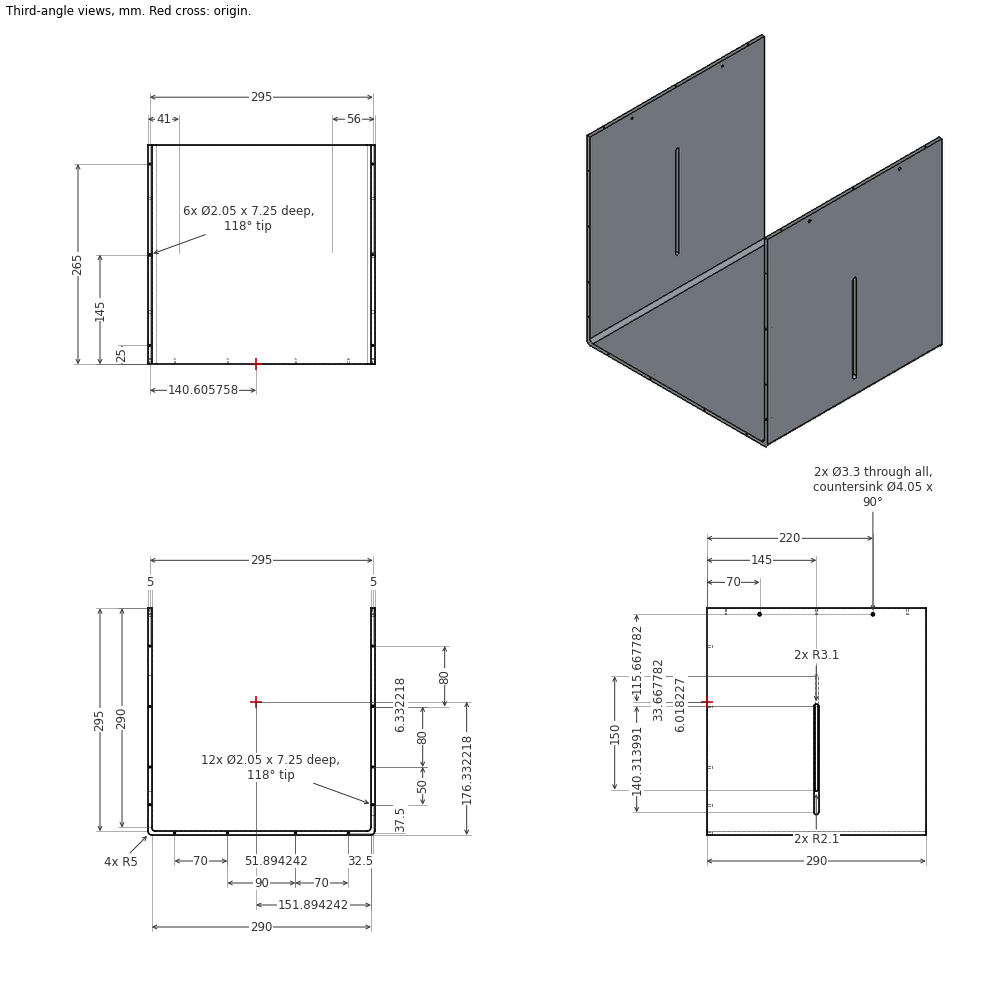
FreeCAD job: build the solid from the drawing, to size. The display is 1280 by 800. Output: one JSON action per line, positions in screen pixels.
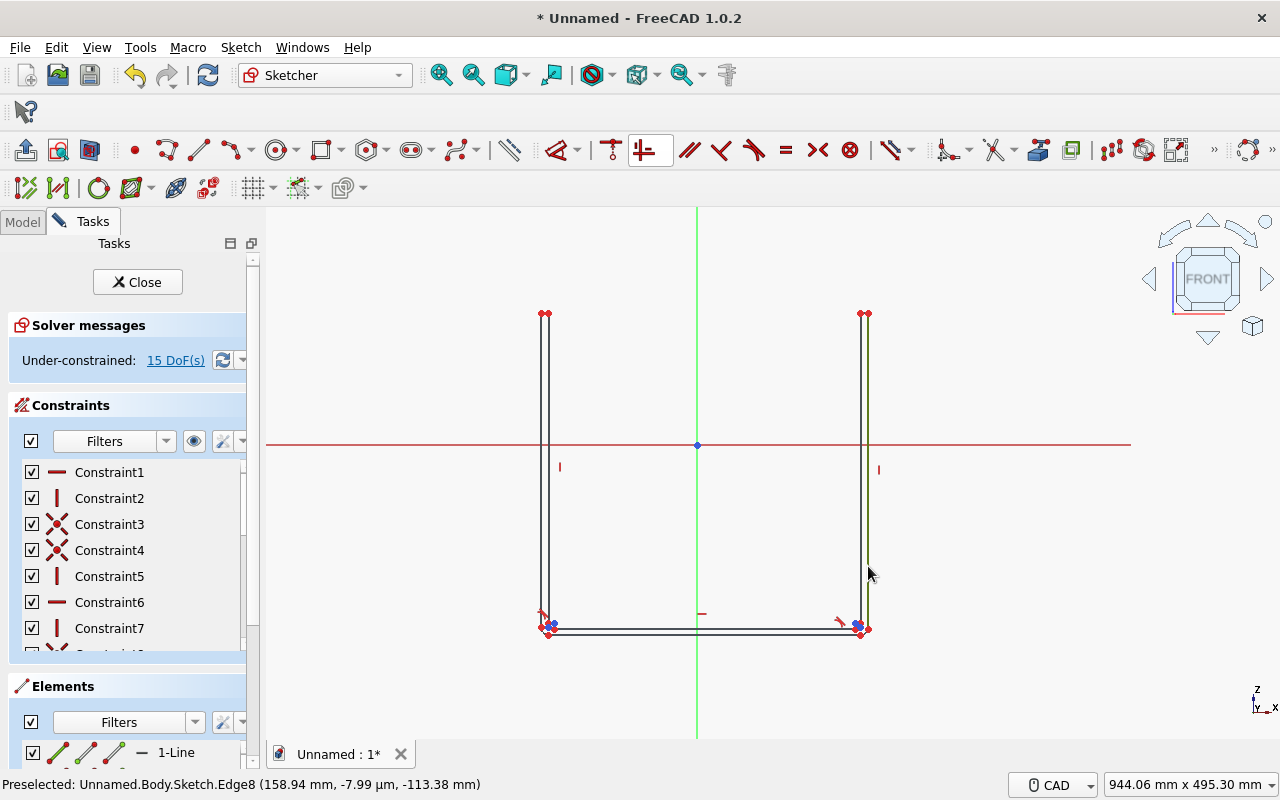
{"action": "scroll", "coordinate": [865, 634], "scroll_direction": "up", "scroll_amount": 5}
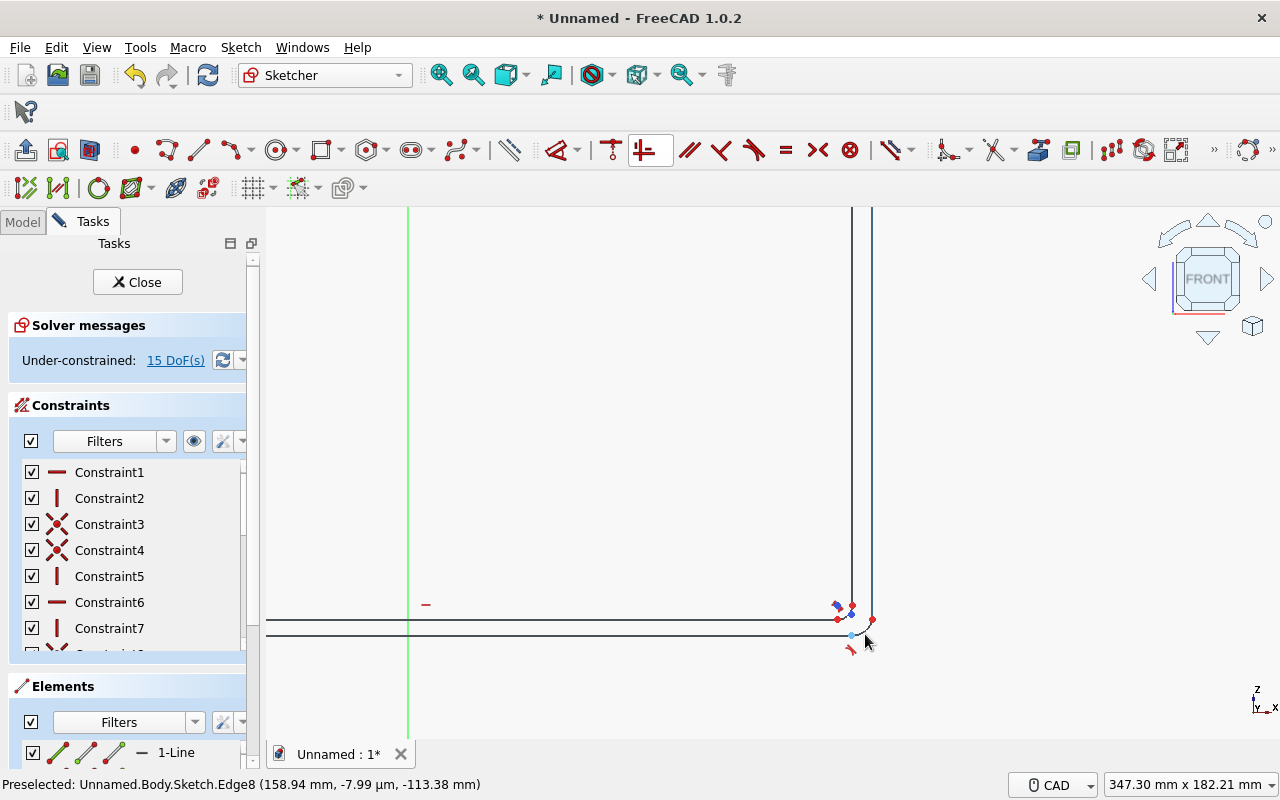
{"action": "left_click", "coordinate": [865, 631]}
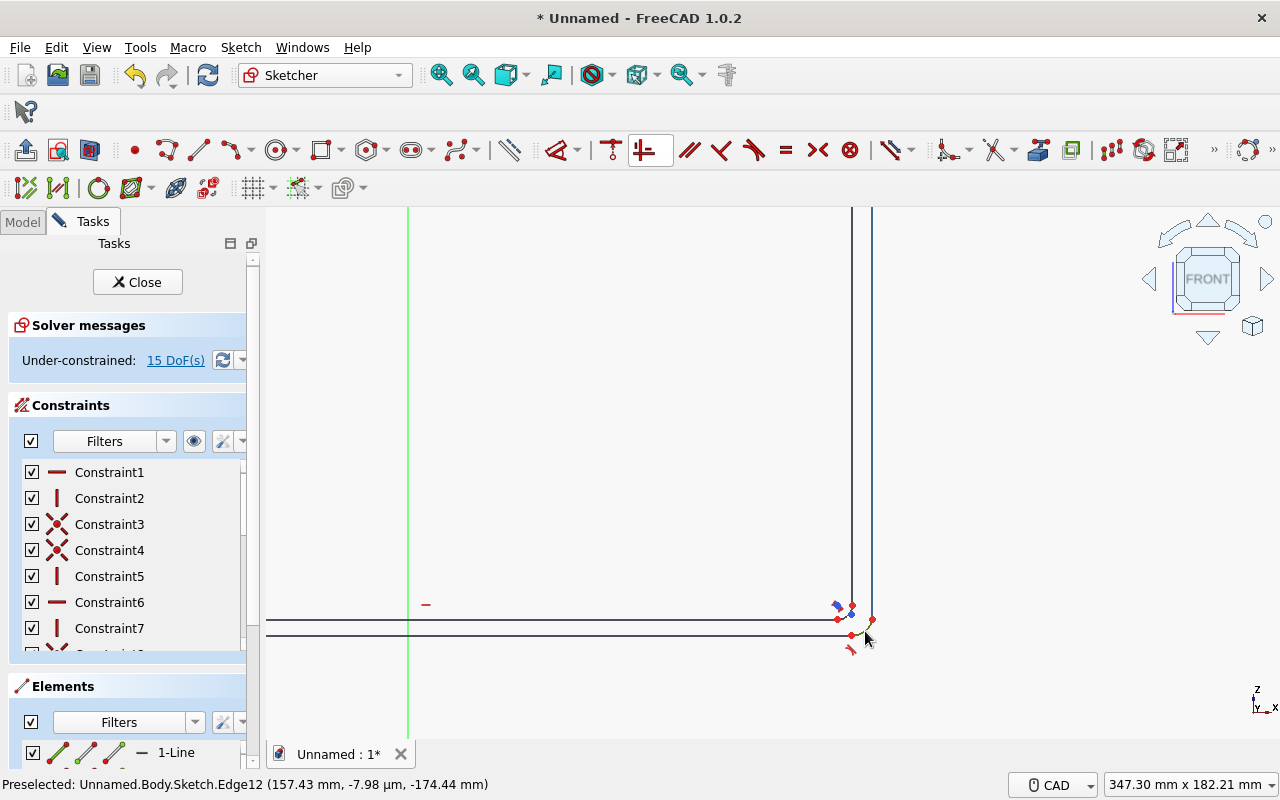
{"action": "left_click", "coordinate": [754, 150]}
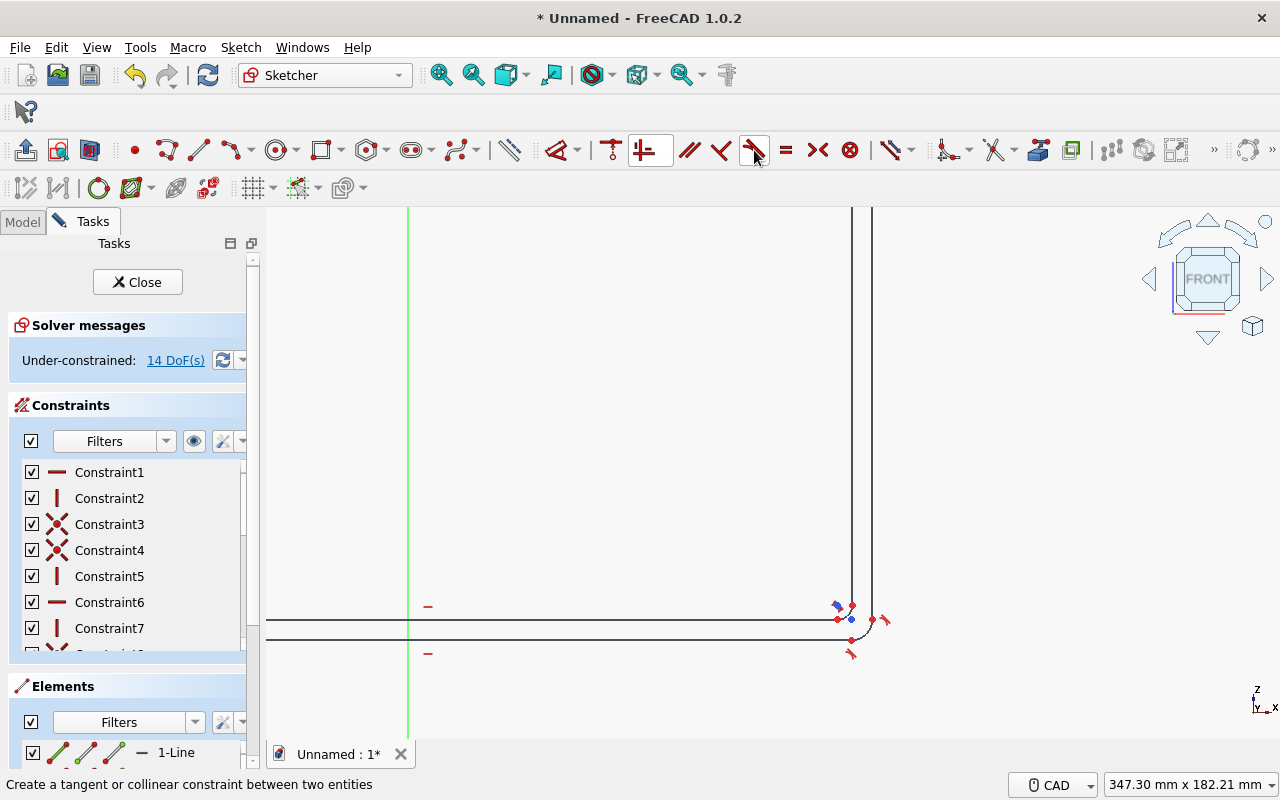
{"action": "scroll", "coordinate": [865, 634], "scroll_direction": "down", "scroll_amount": 5}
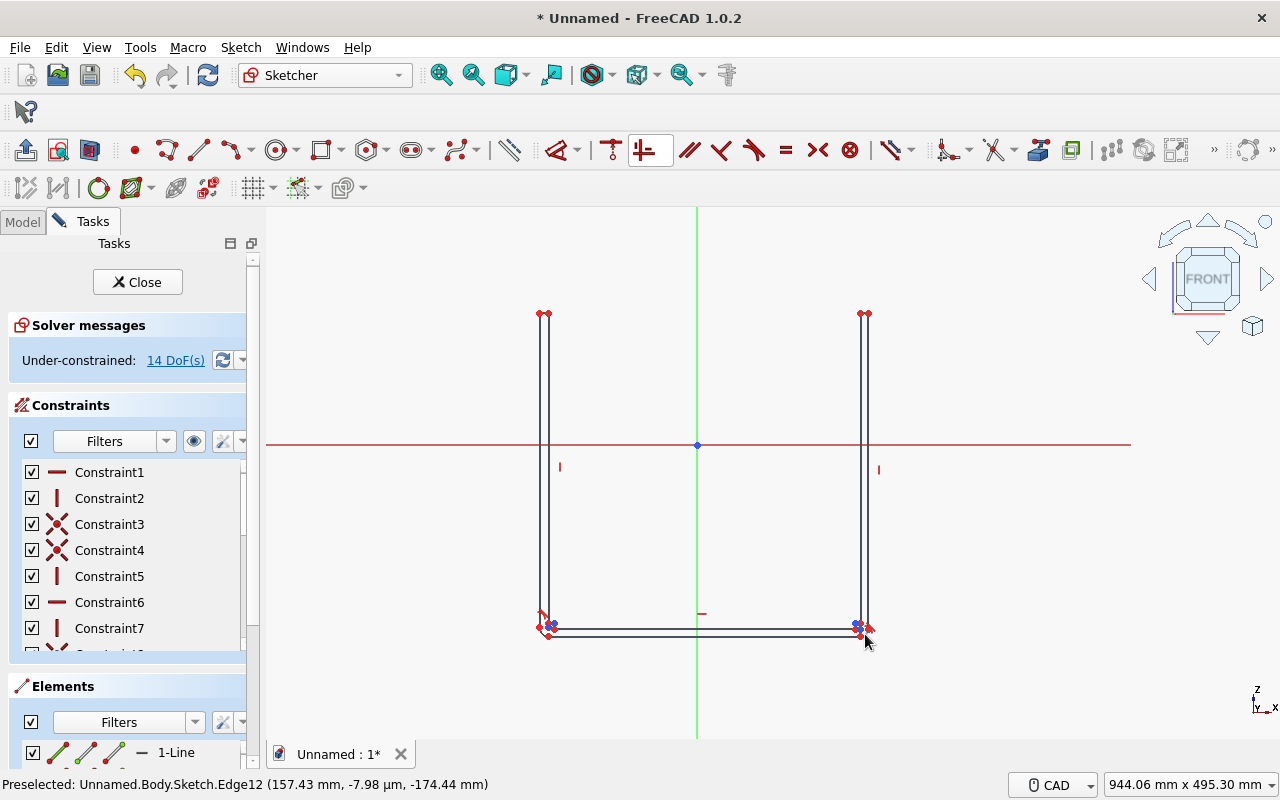
{"action": "scroll", "coordinate": [543, 313], "scroll_direction": "up", "scroll_amount": 7}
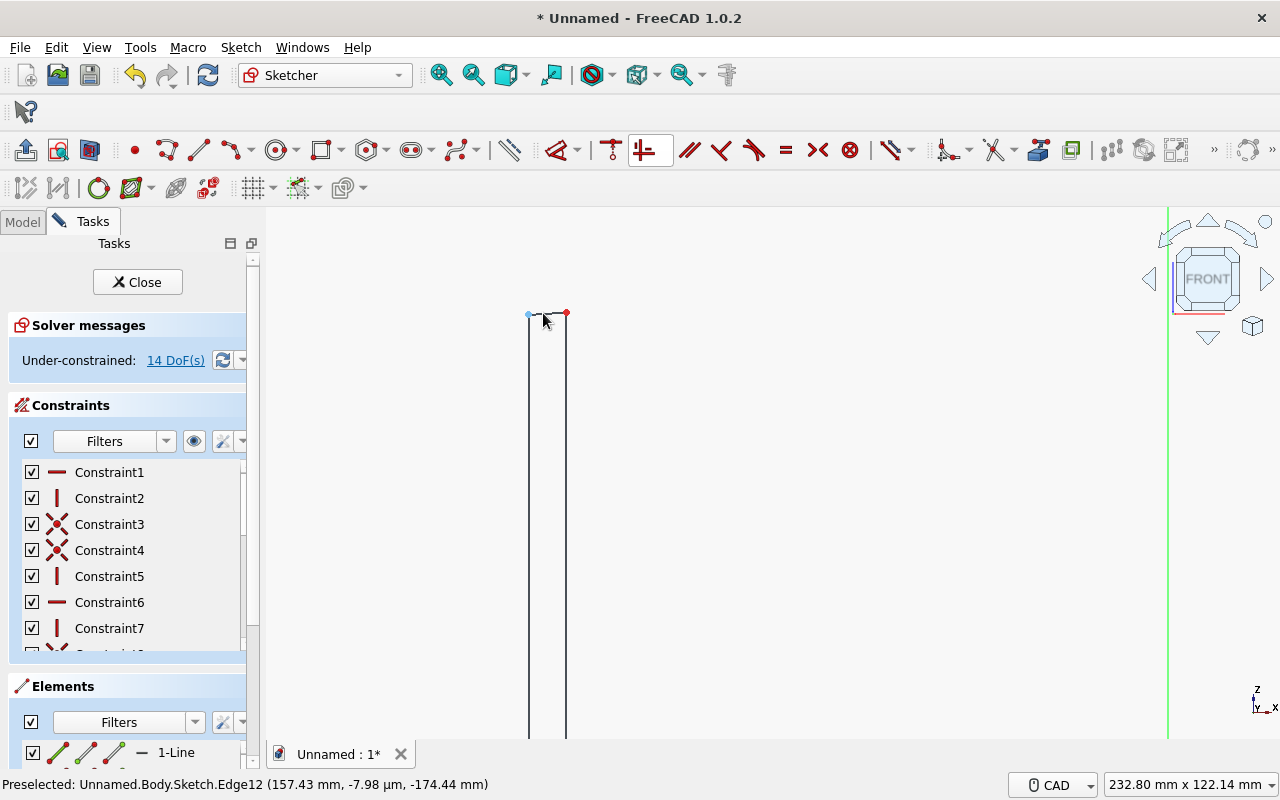
{"action": "left_click", "coordinate": [544, 314]}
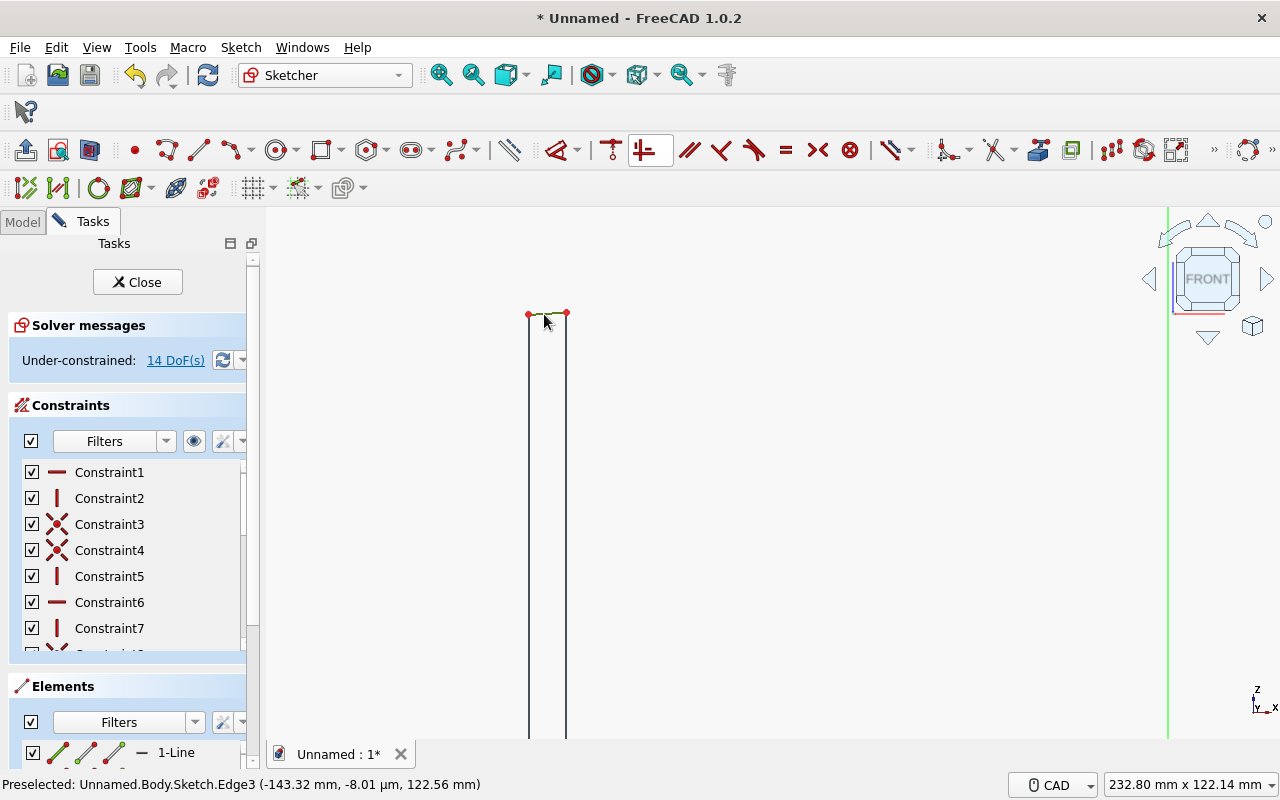
{"action": "left_click", "coordinate": [668, 150]}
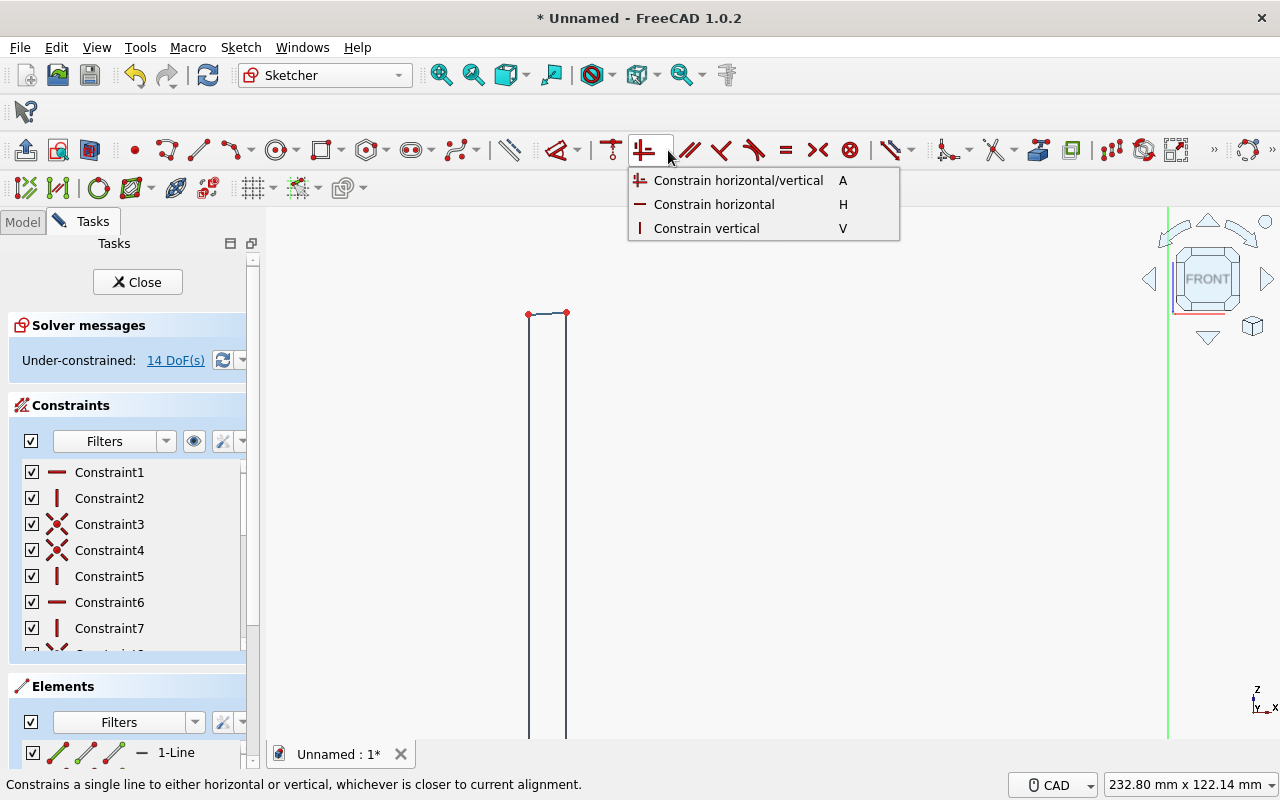
{"action": "left_click", "coordinate": [764, 204]}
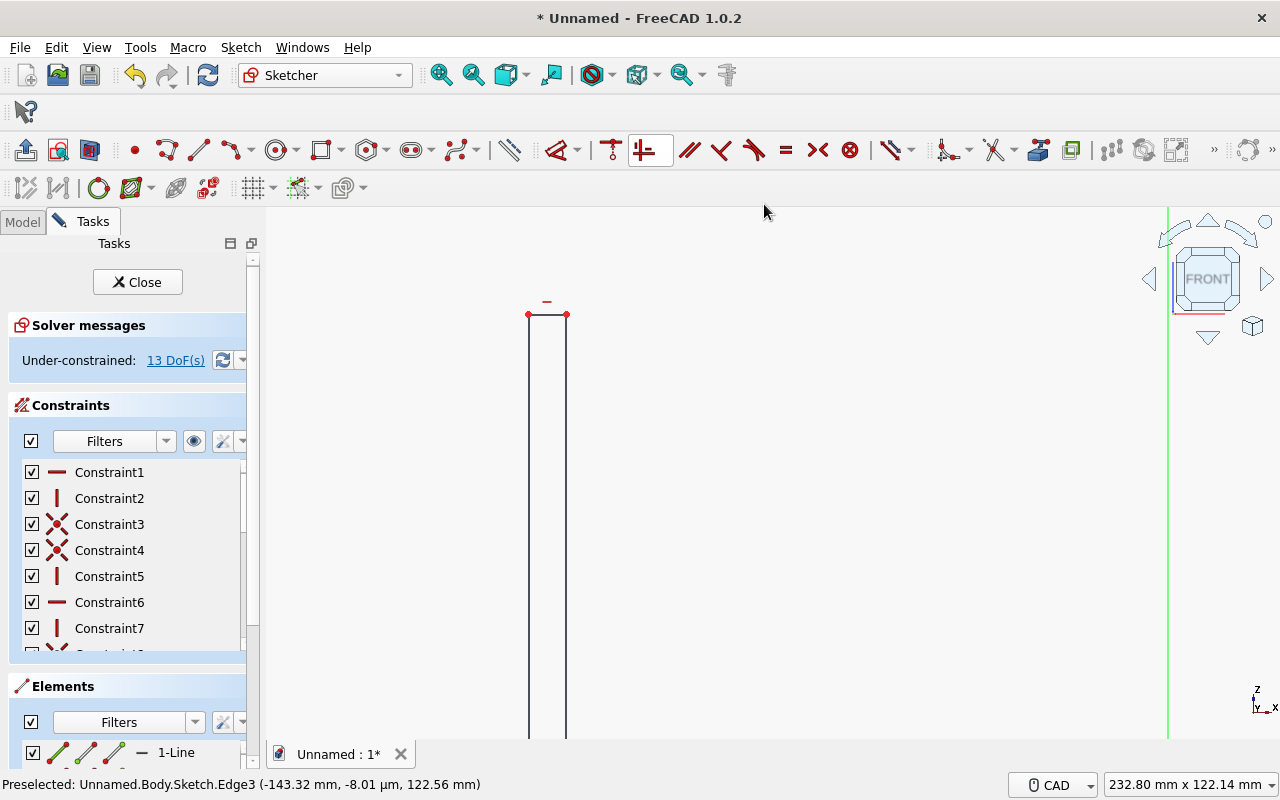
{"action": "scroll", "coordinate": [543, 313], "scroll_direction": "down", "scroll_amount": 7}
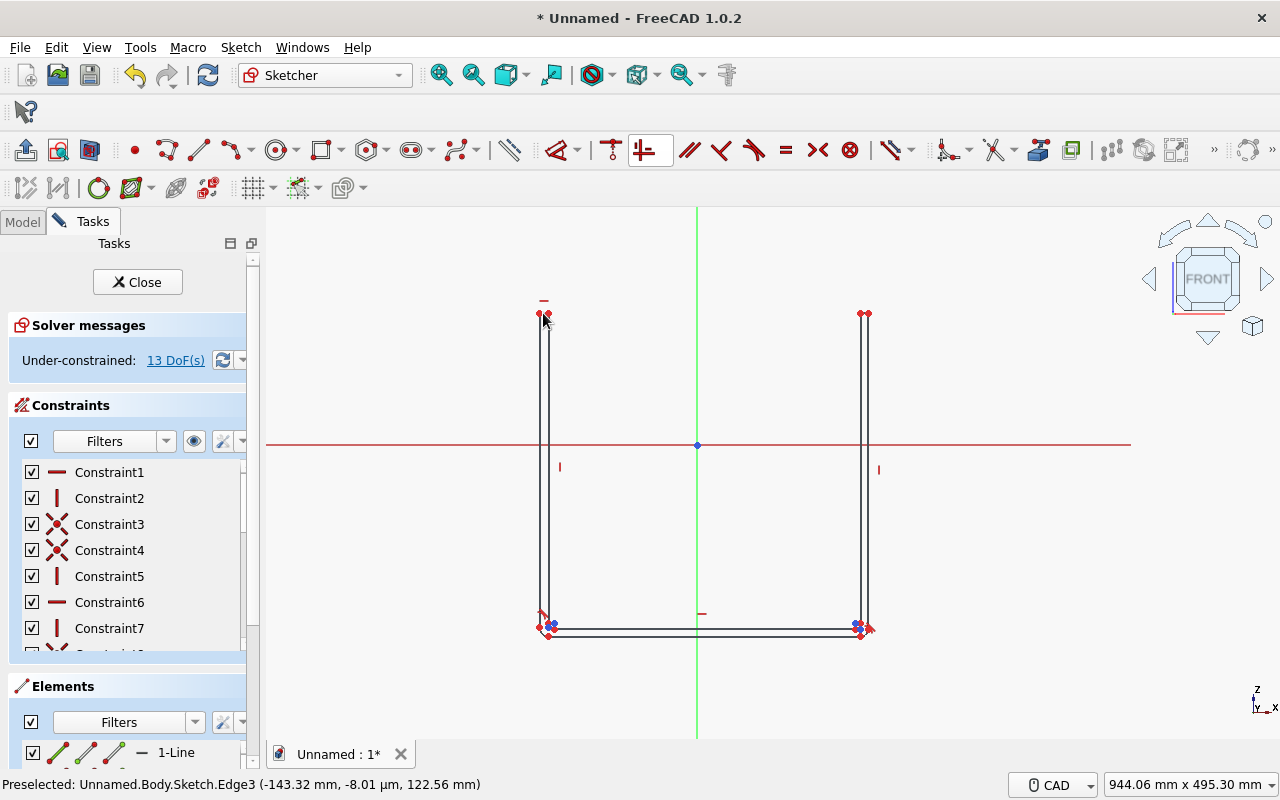
{"action": "scroll", "coordinate": [863, 313], "scroll_direction": "up", "scroll_amount": 10}